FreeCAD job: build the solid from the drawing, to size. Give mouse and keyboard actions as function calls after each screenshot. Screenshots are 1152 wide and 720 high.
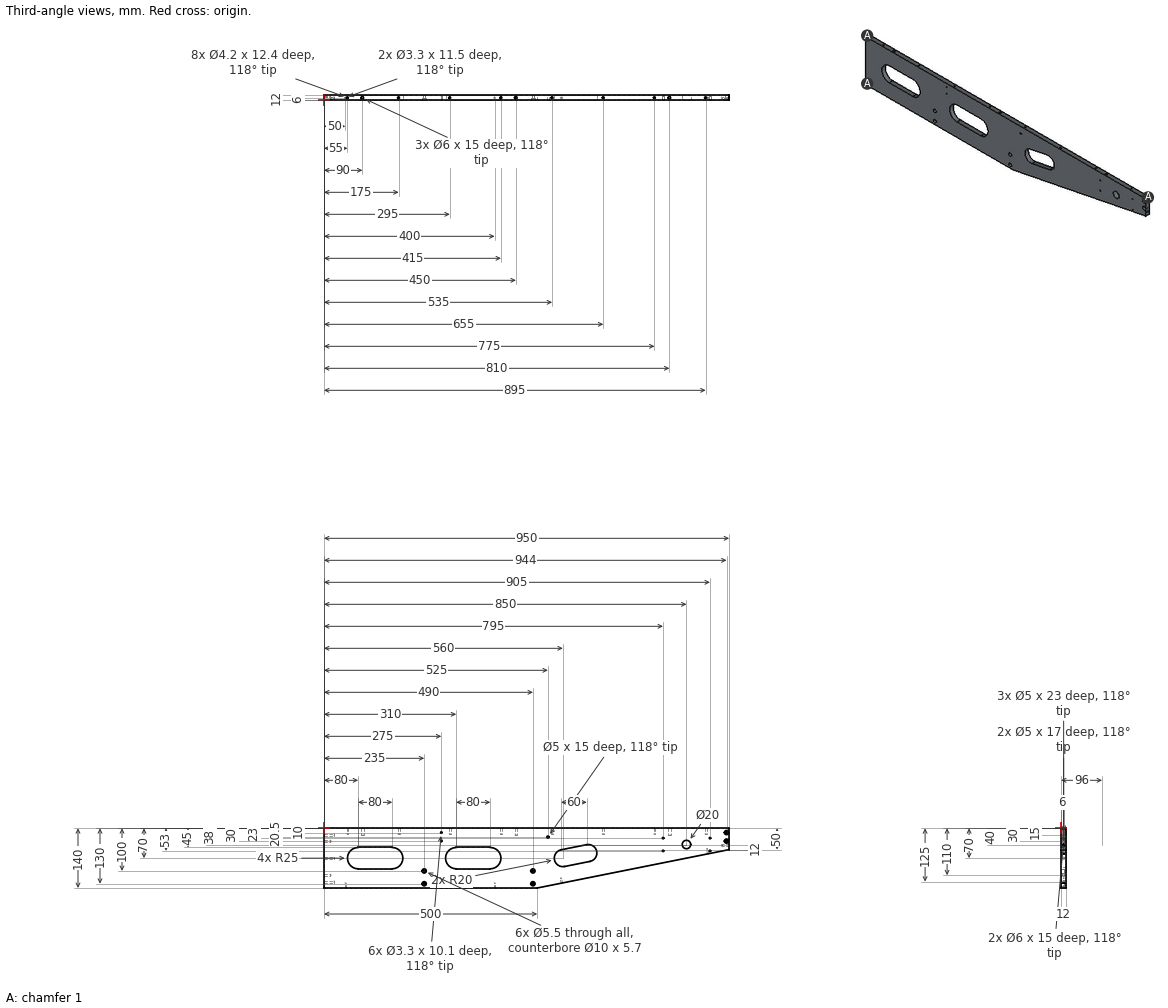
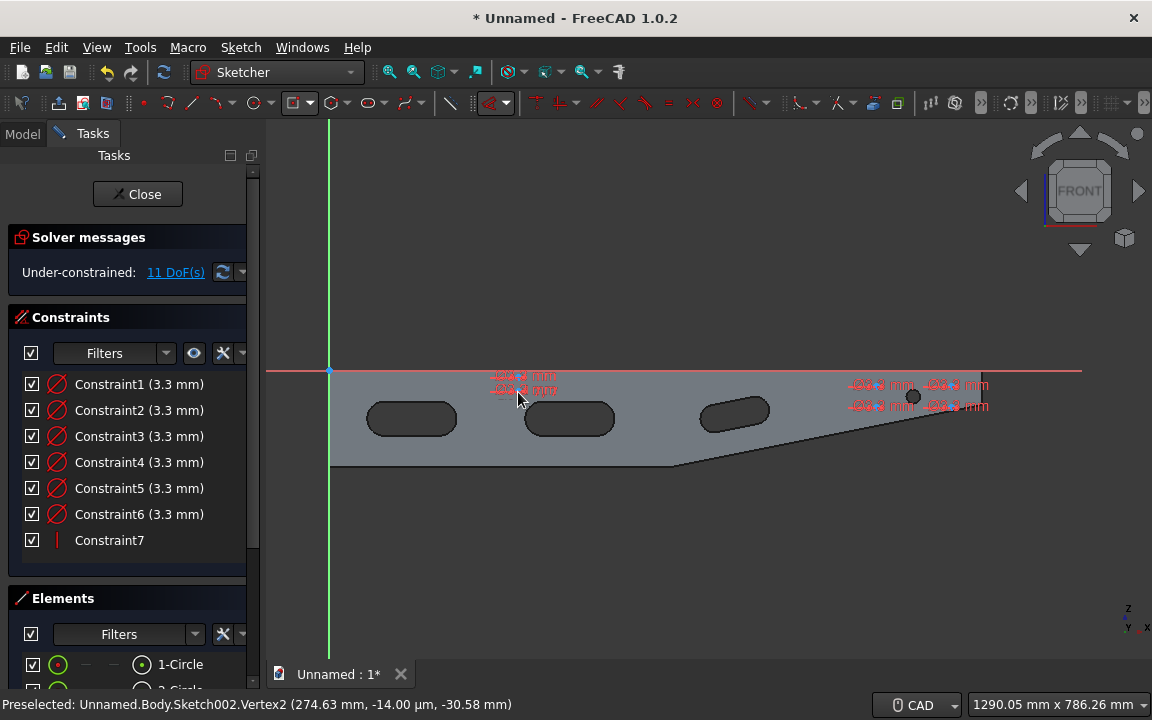
click(876, 387)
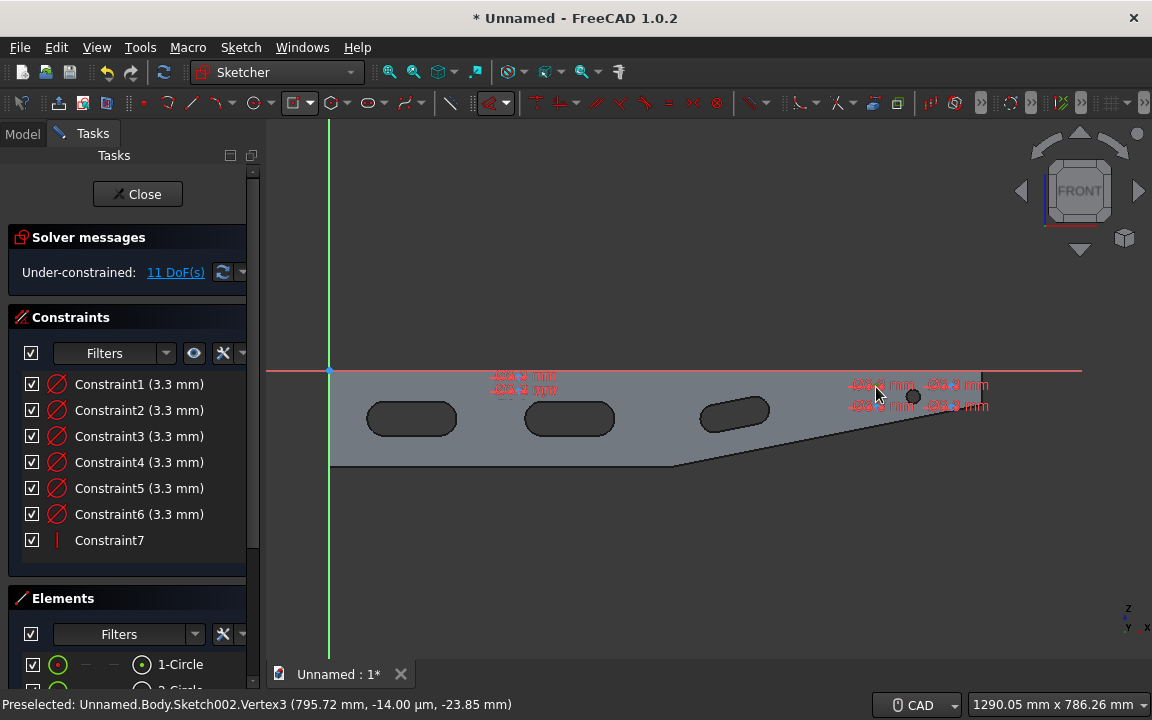
click(951, 387)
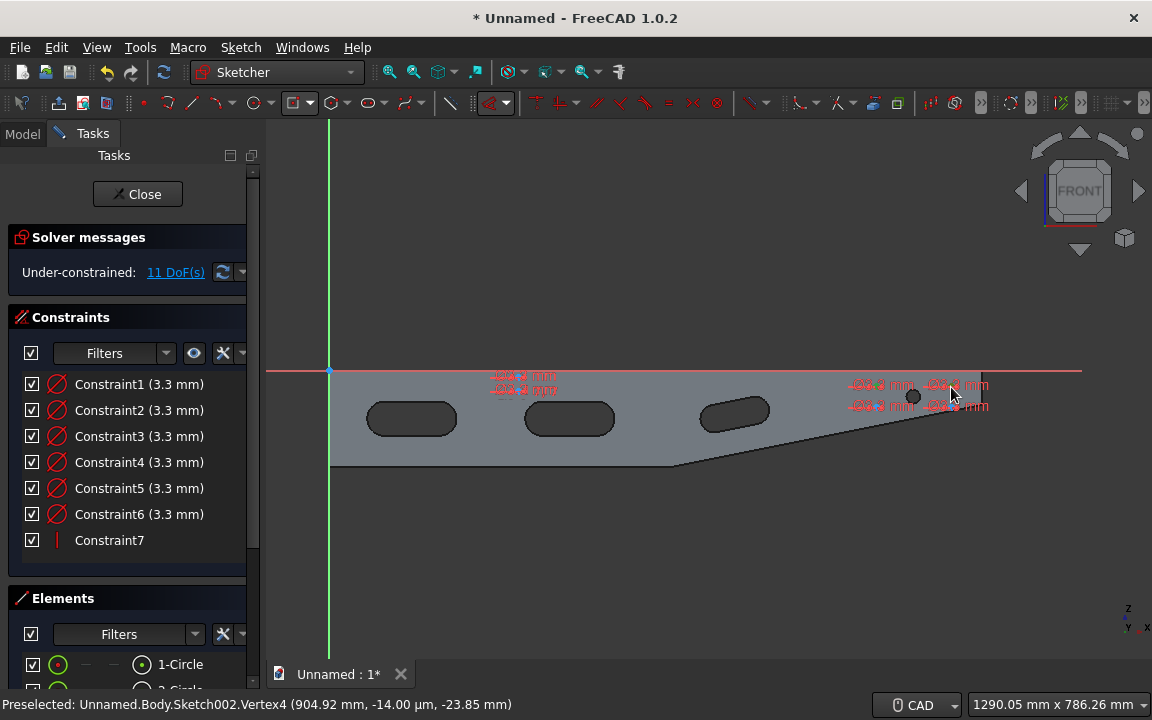
key(h)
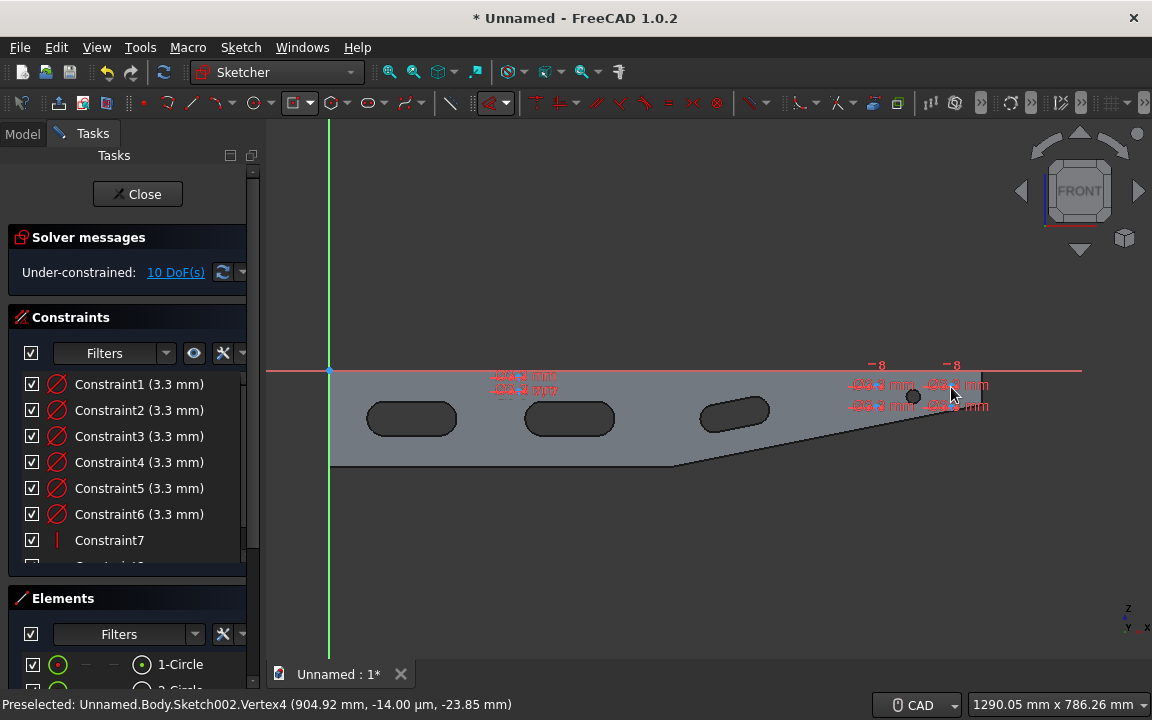
click(876, 387)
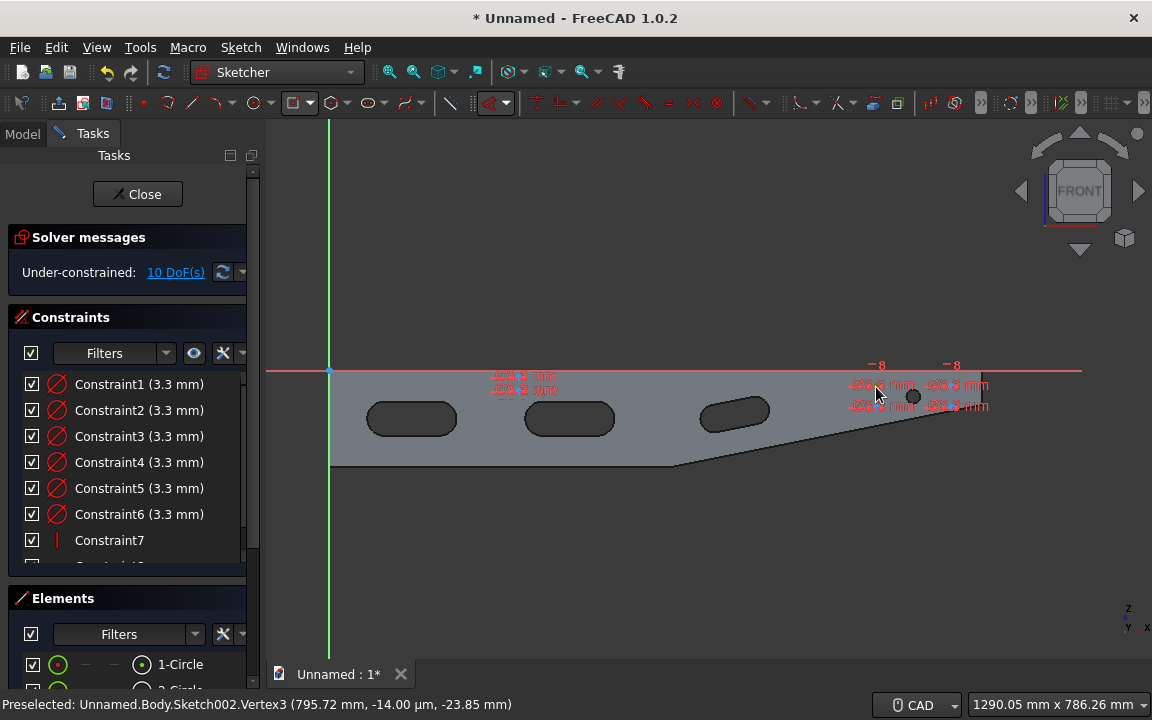
click(876, 408)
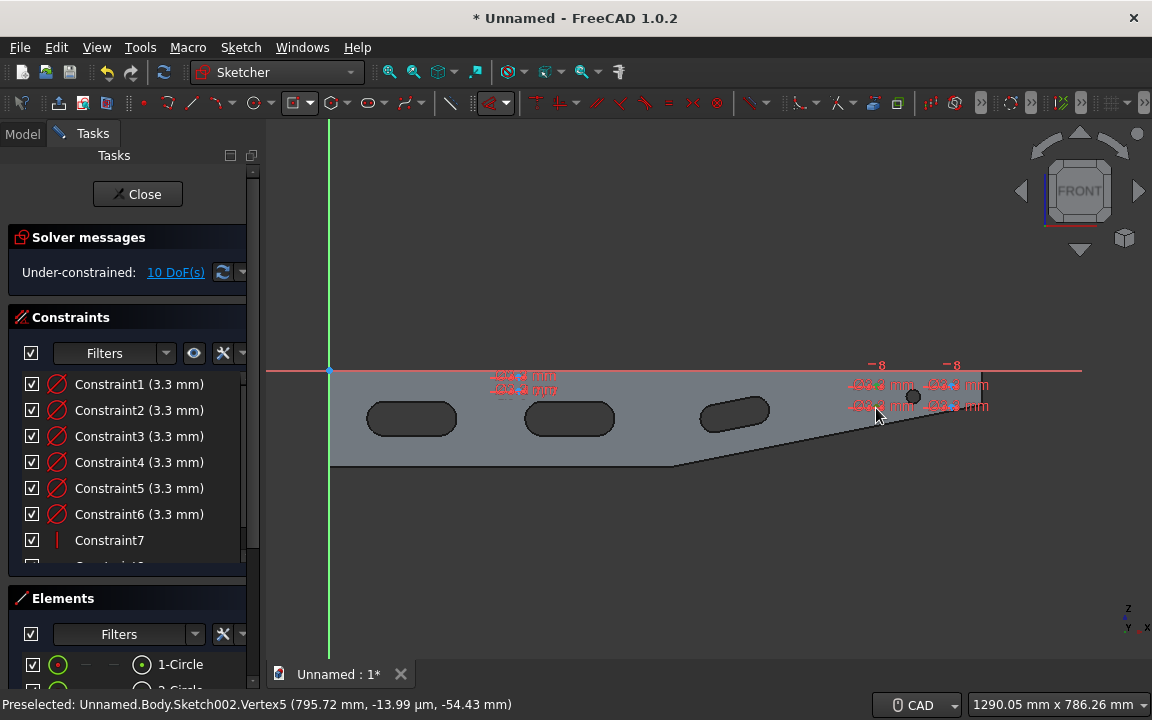
key(v)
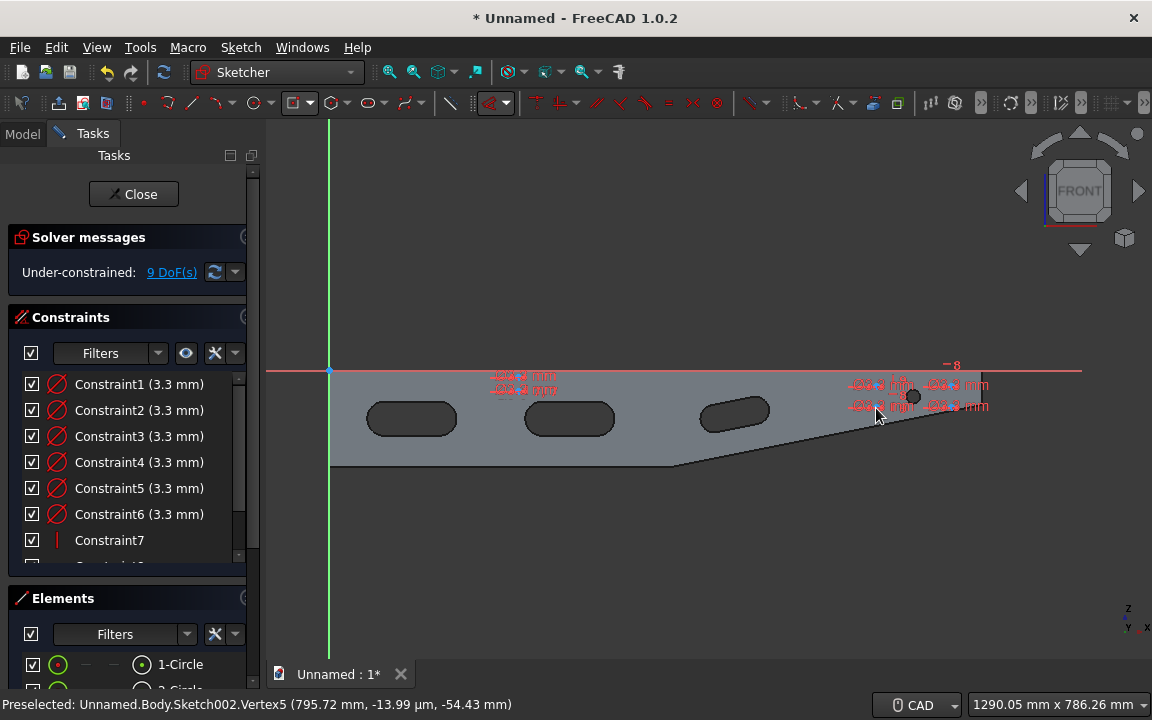
click(951, 387)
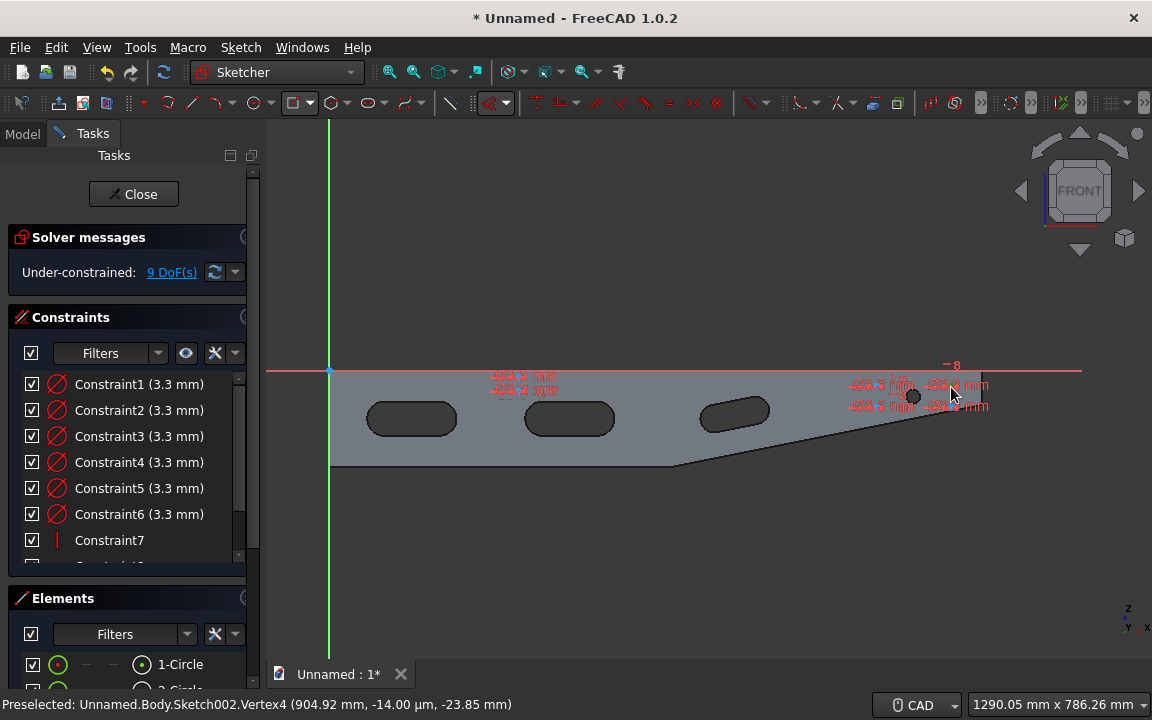
click(951, 408)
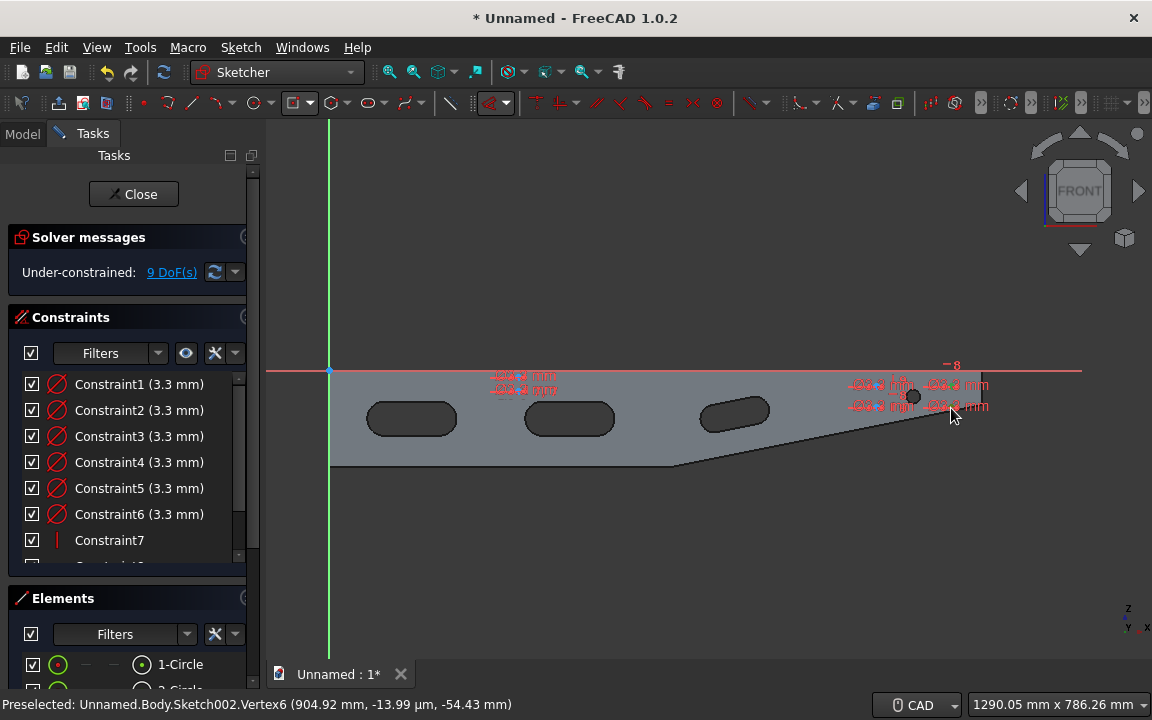
key(v)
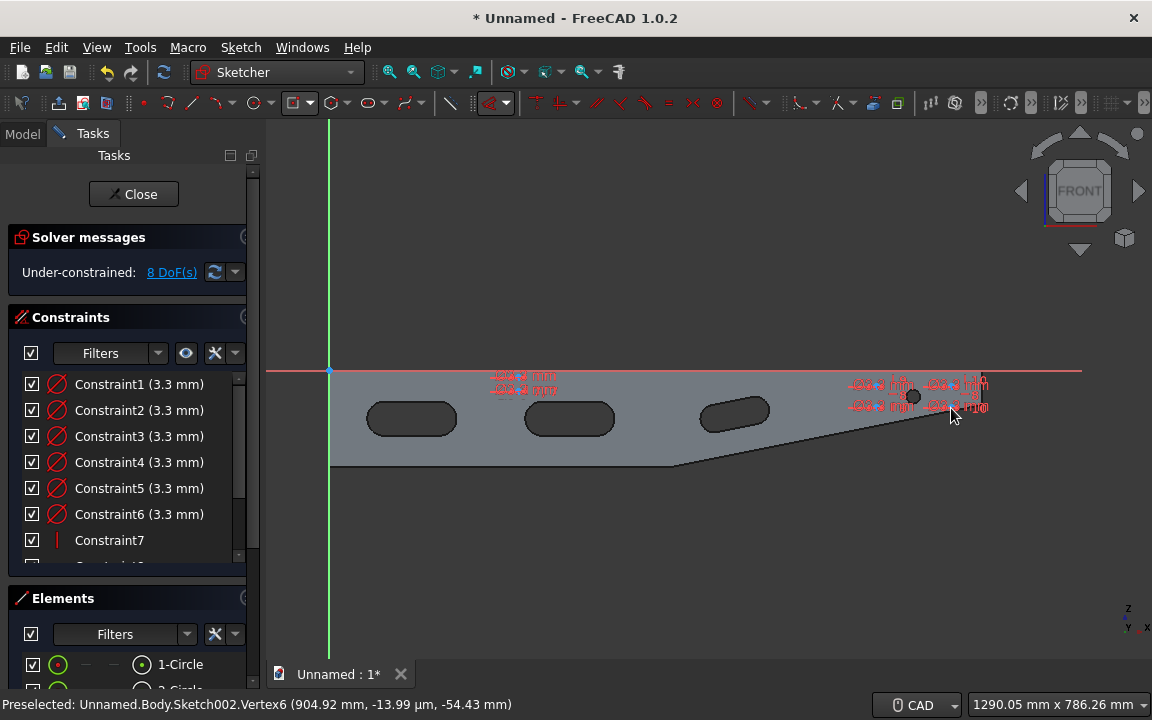
click(876, 408)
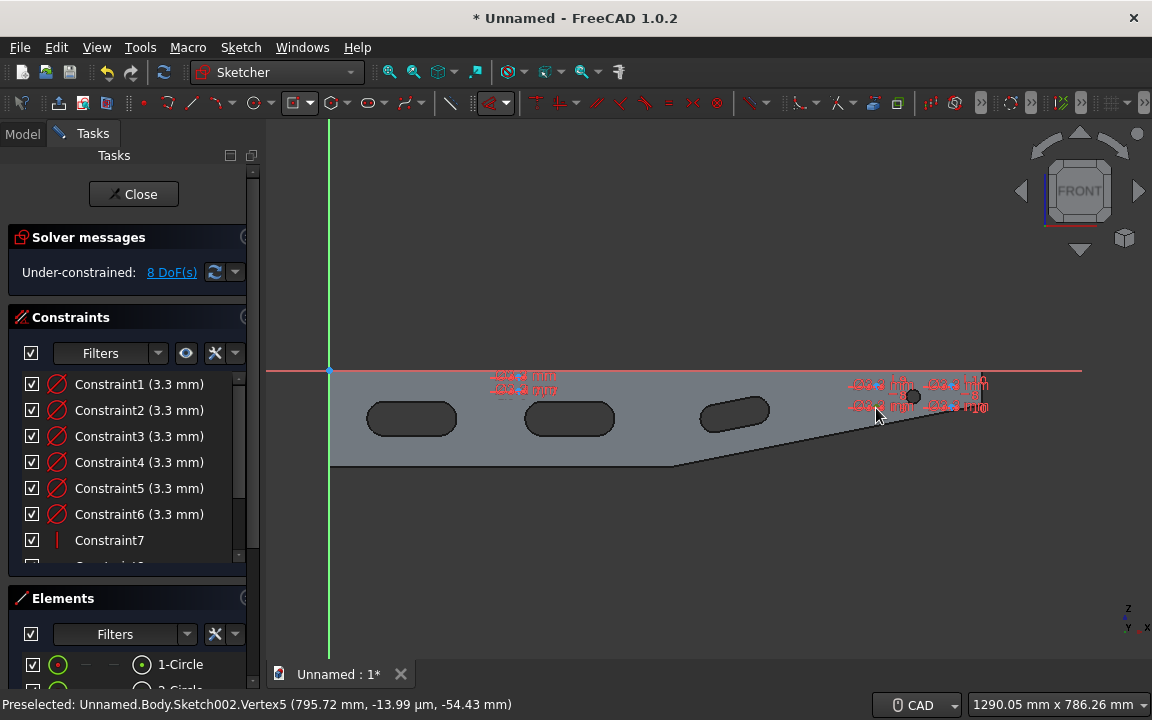
click(951, 408)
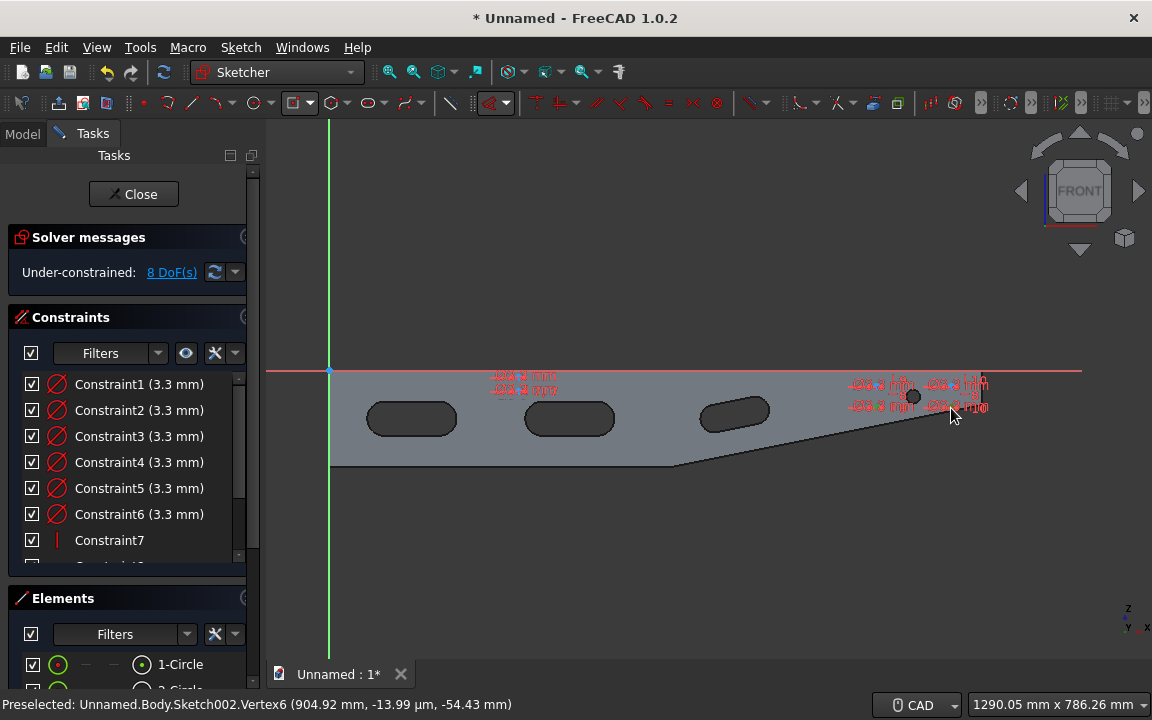
key(h)